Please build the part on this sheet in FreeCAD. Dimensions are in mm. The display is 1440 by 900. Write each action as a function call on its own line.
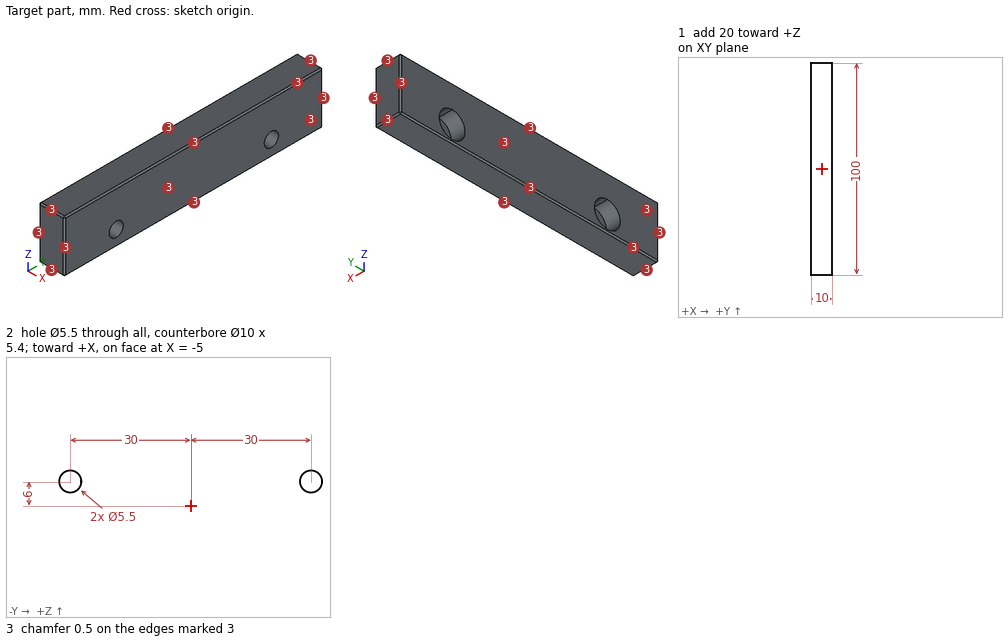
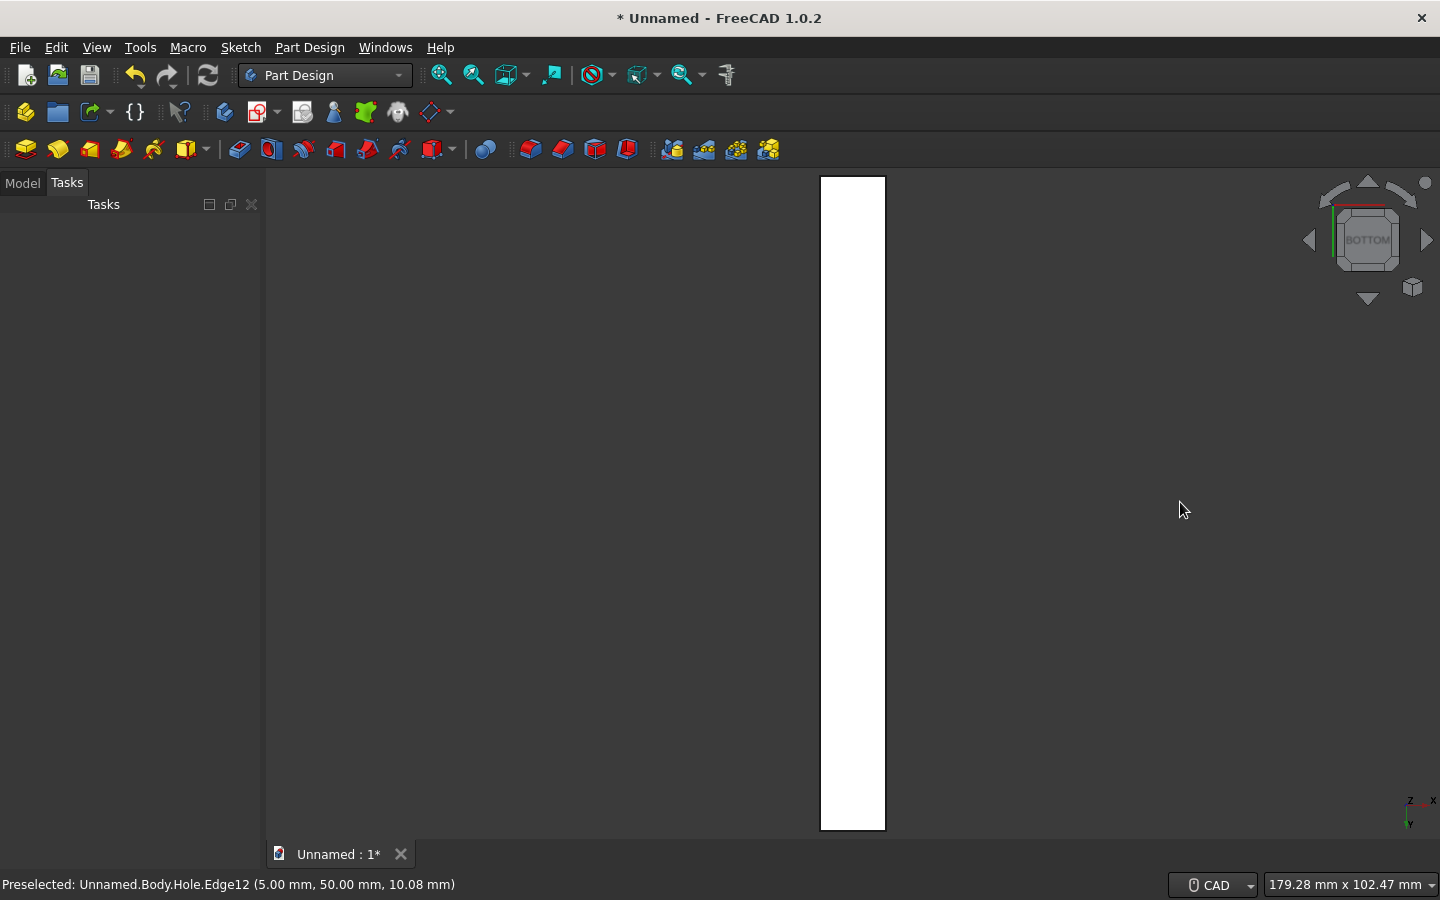
click(853, 783, ctrl)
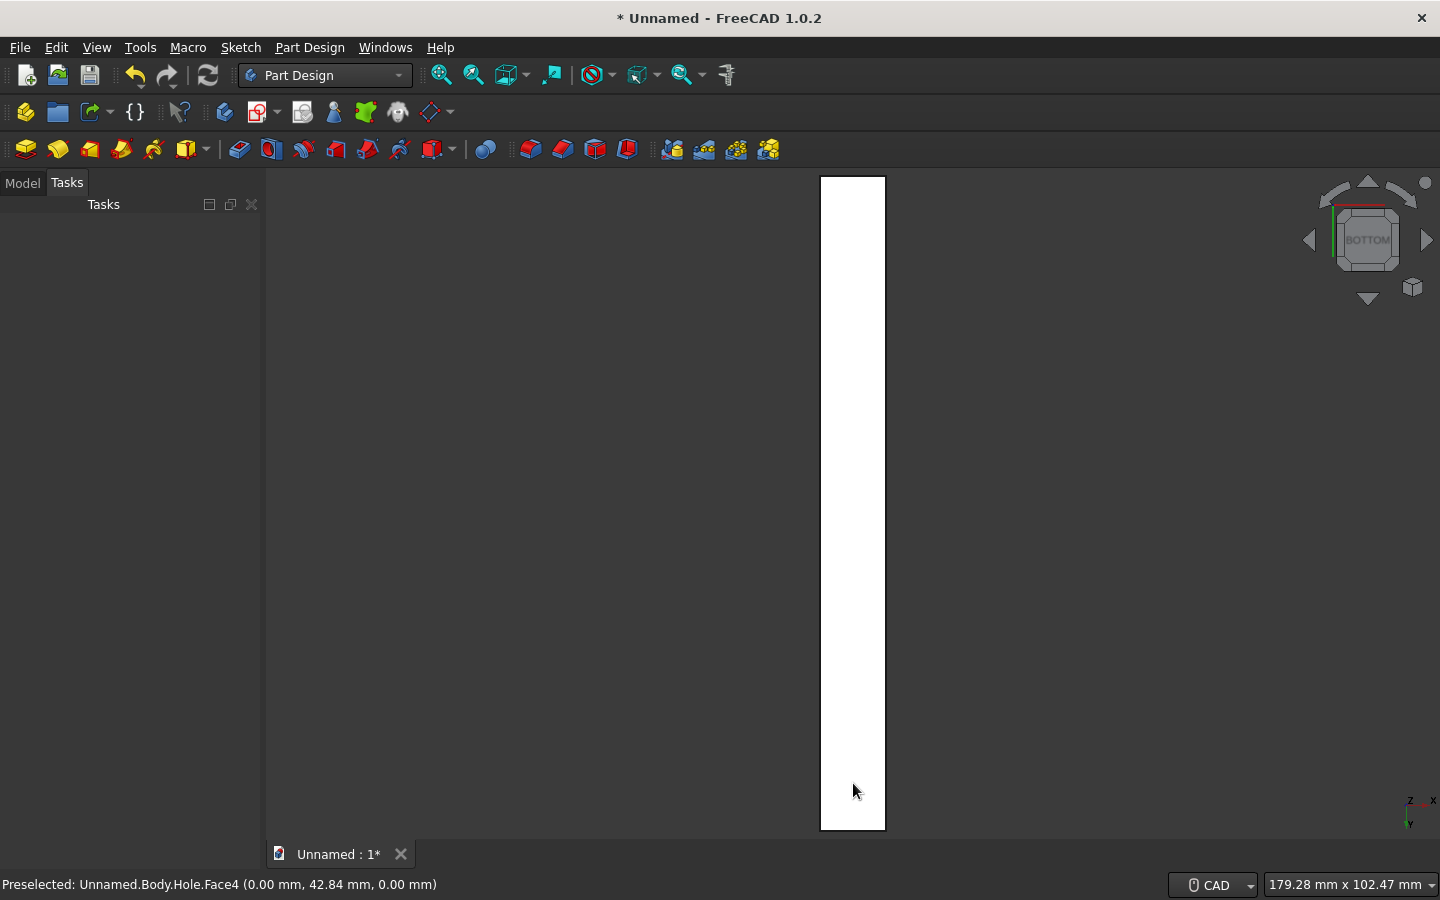
click(564, 150)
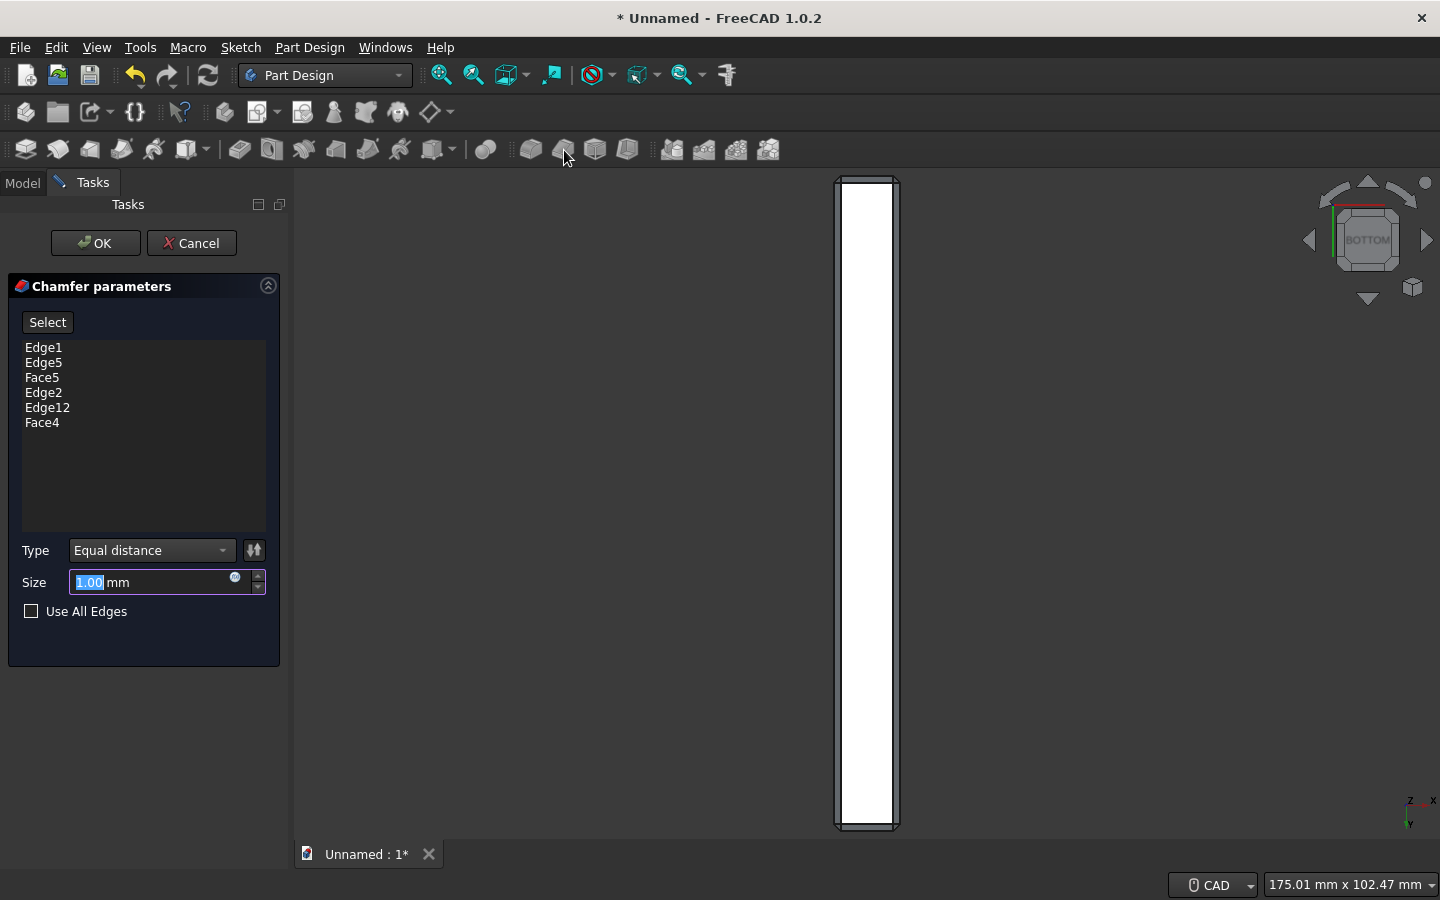
text(0.5)
key(Tab)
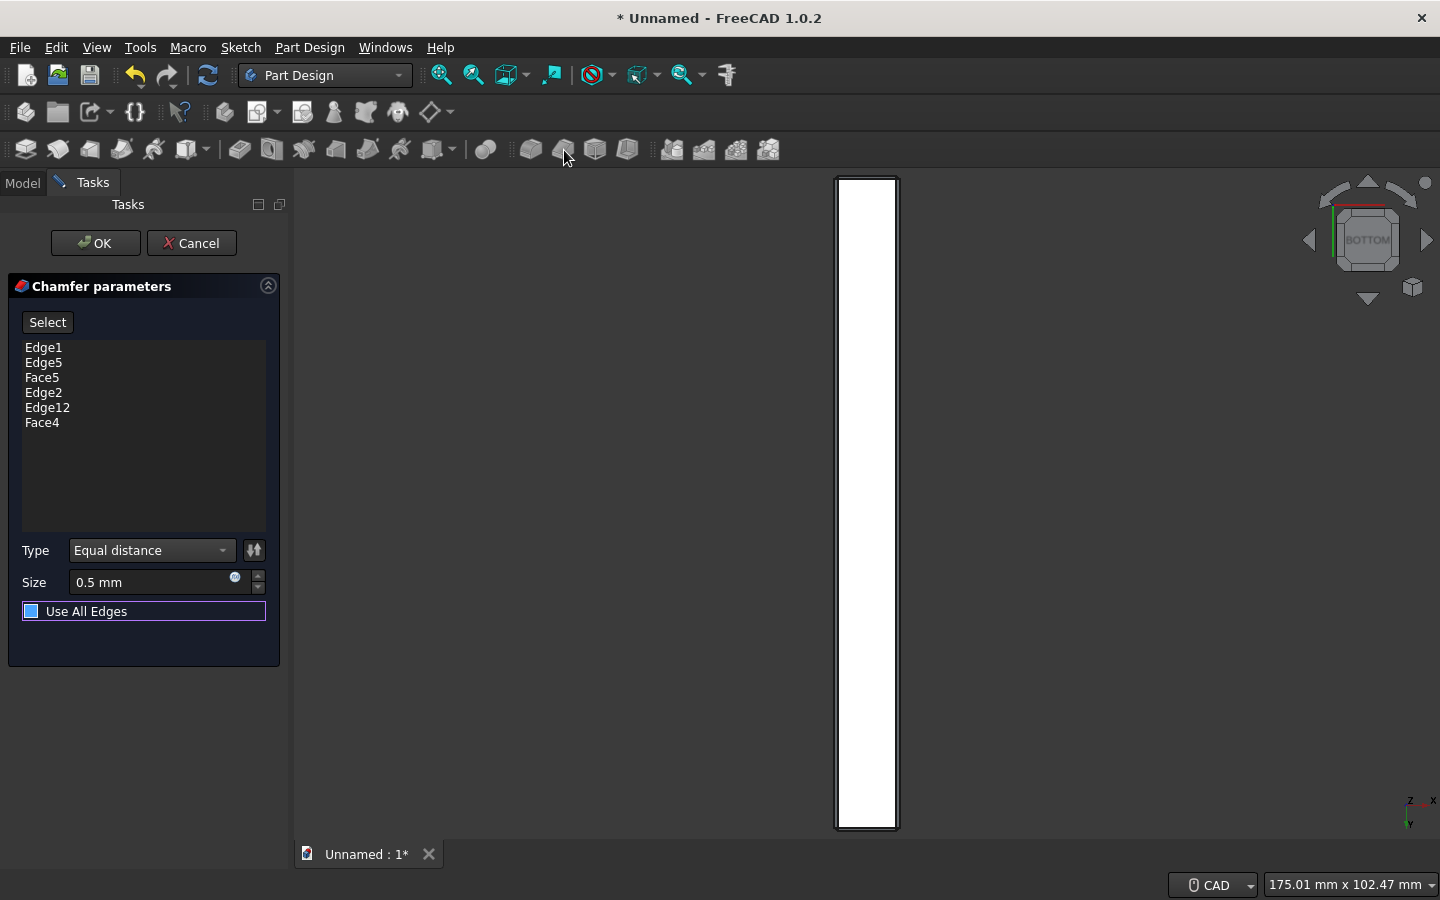
click(96, 243)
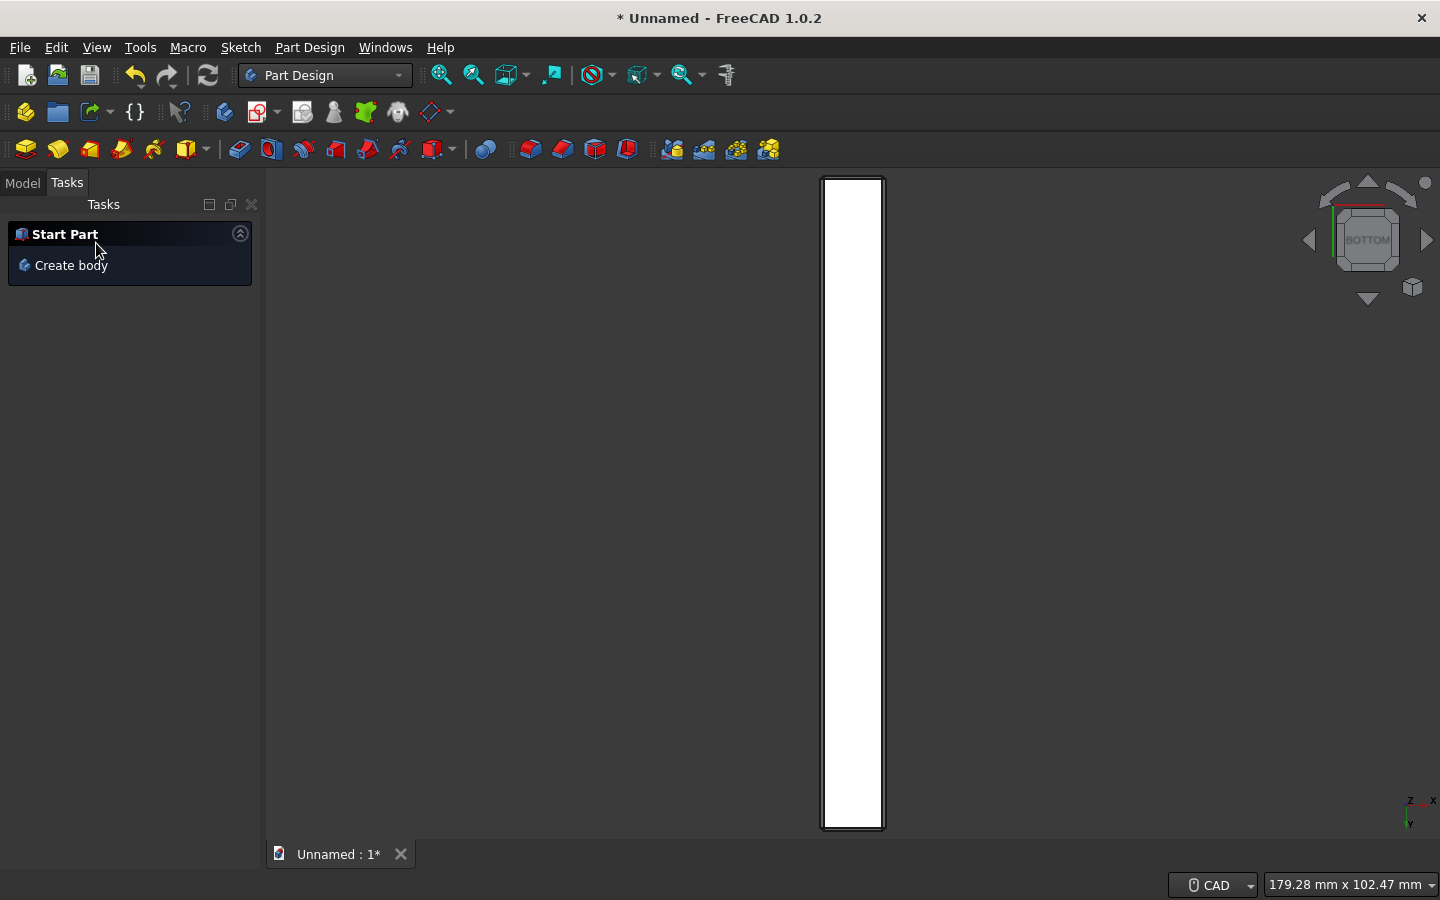
key(0)